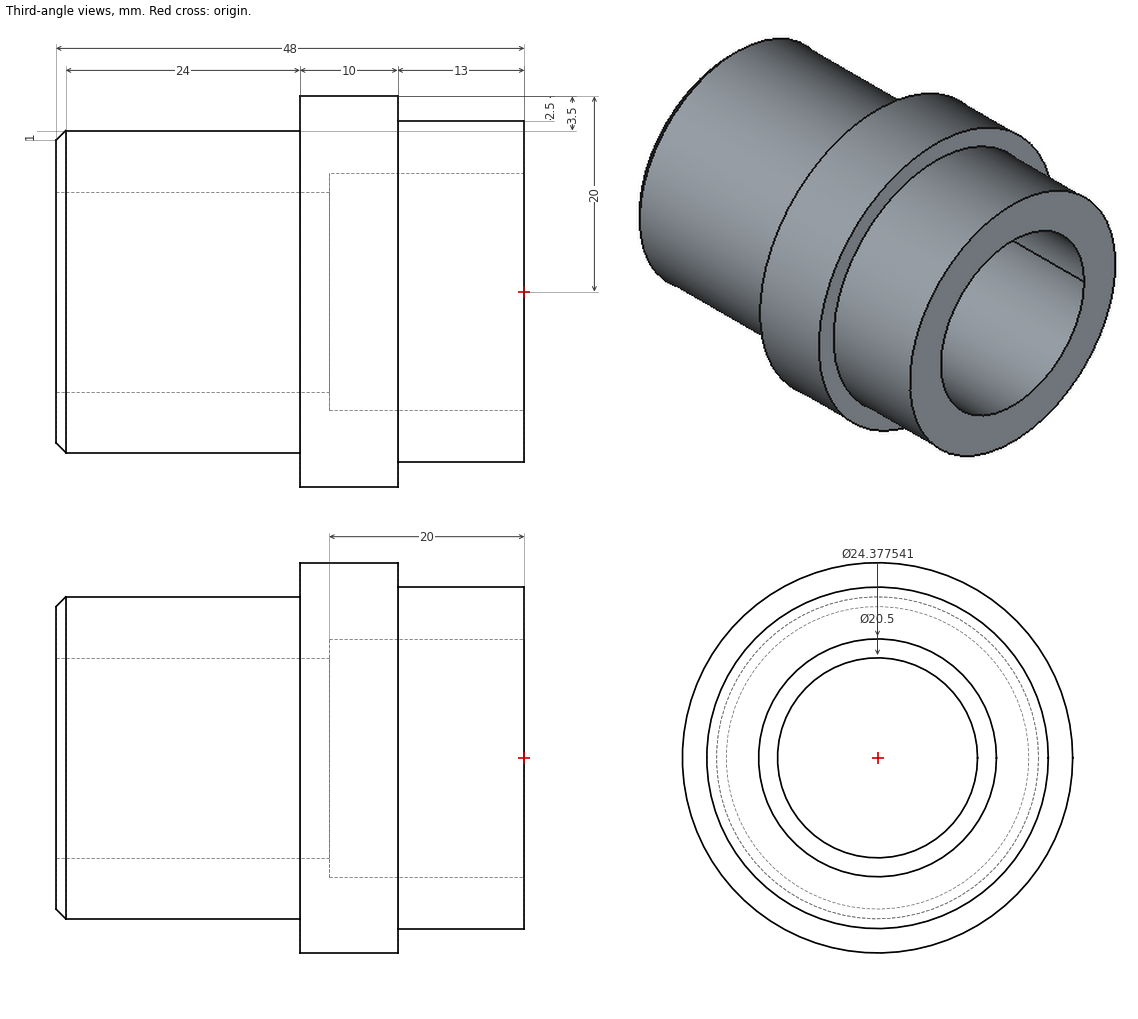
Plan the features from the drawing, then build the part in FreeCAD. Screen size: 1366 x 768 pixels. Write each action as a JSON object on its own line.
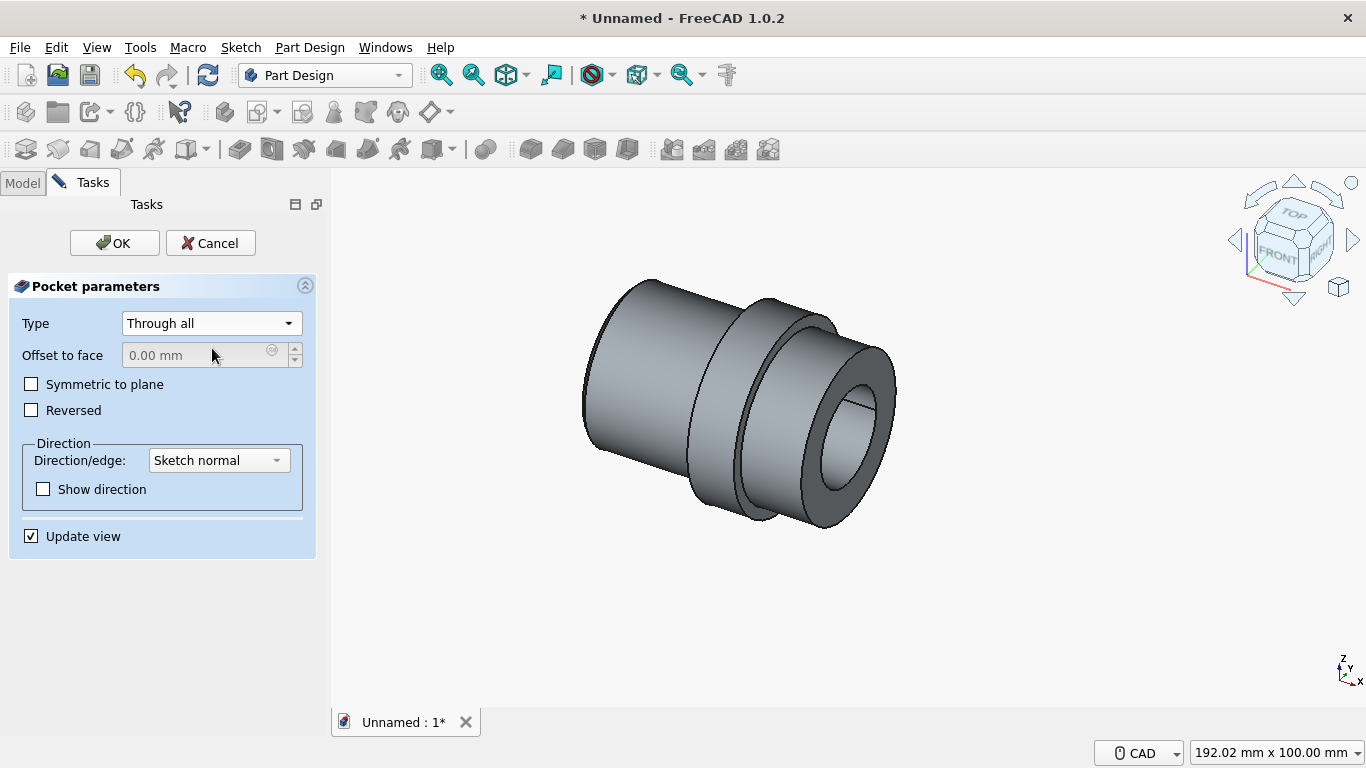
{"action": "left_click", "coordinate": [115, 243]}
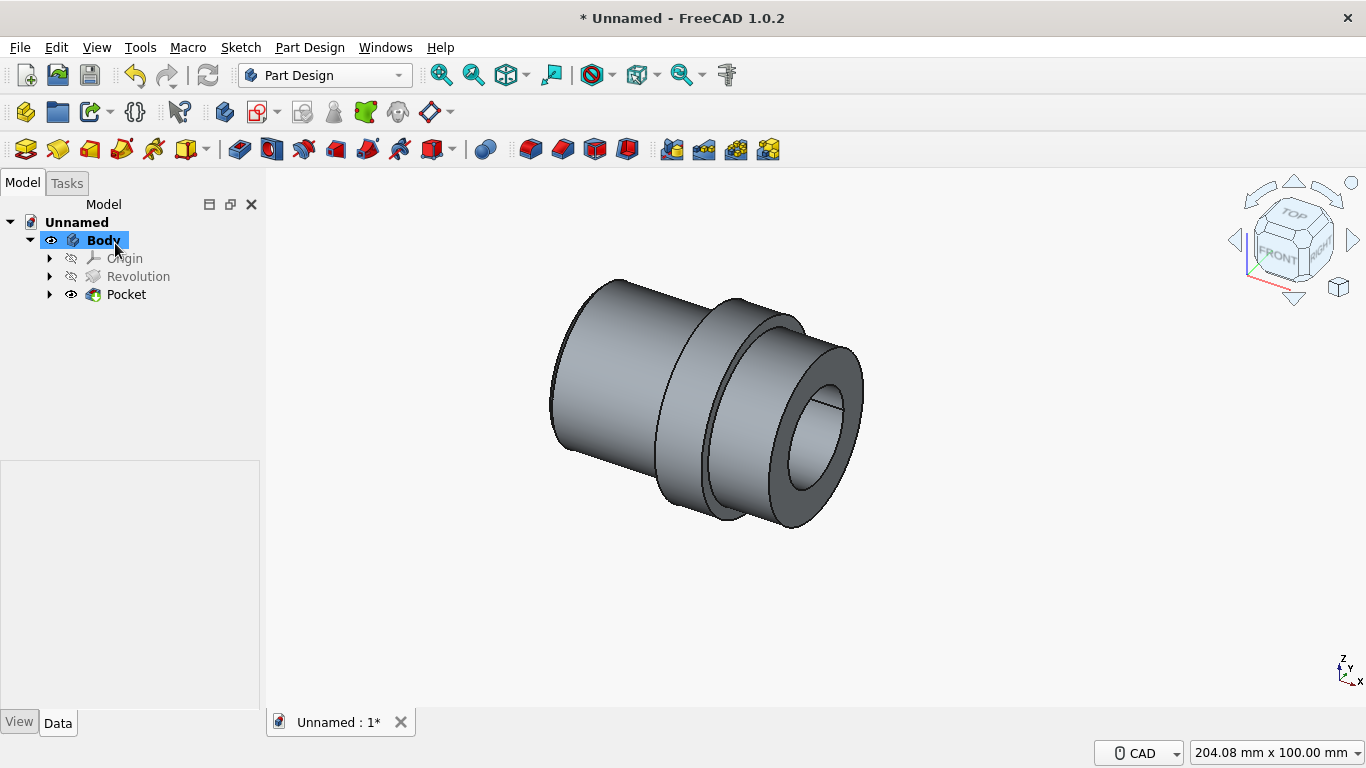
{"action": "left_click", "coordinate": [789, 507]}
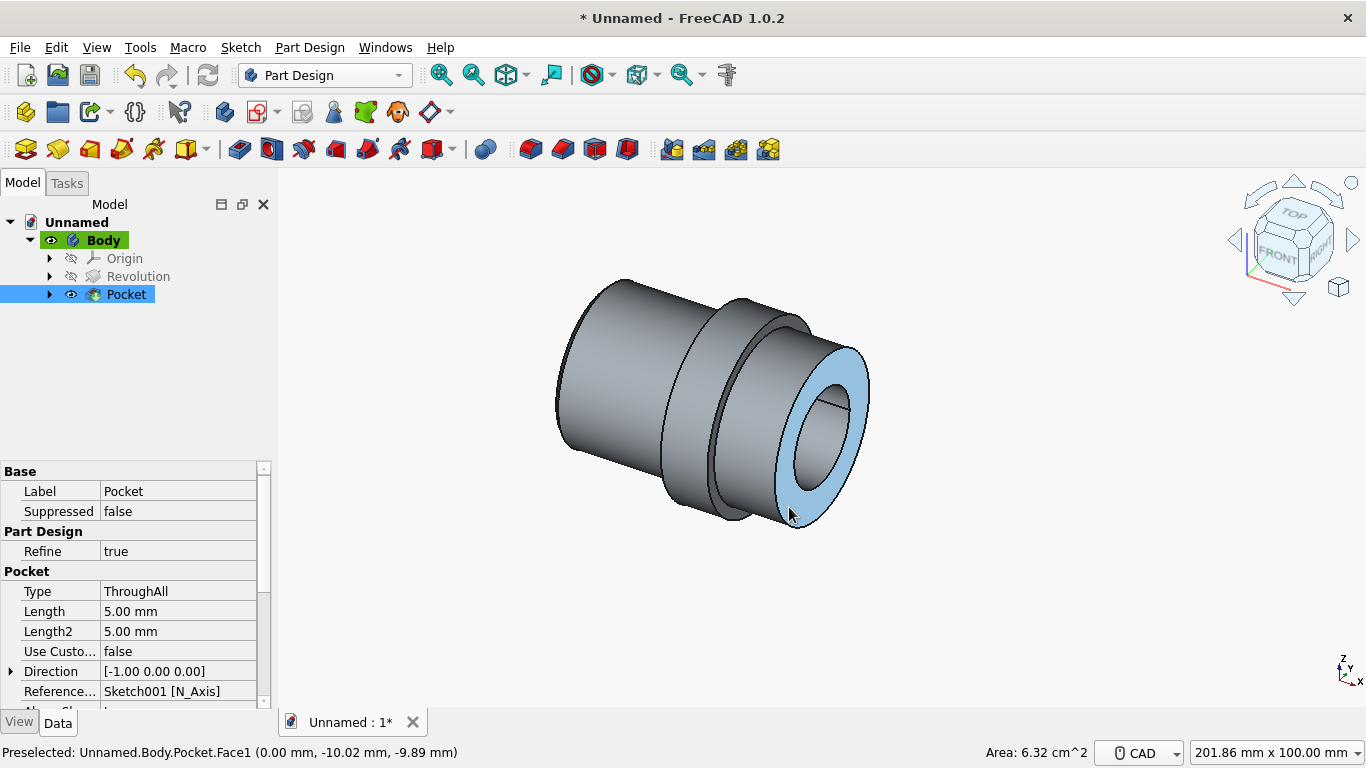
{"action": "left_click", "coordinate": [258, 112]}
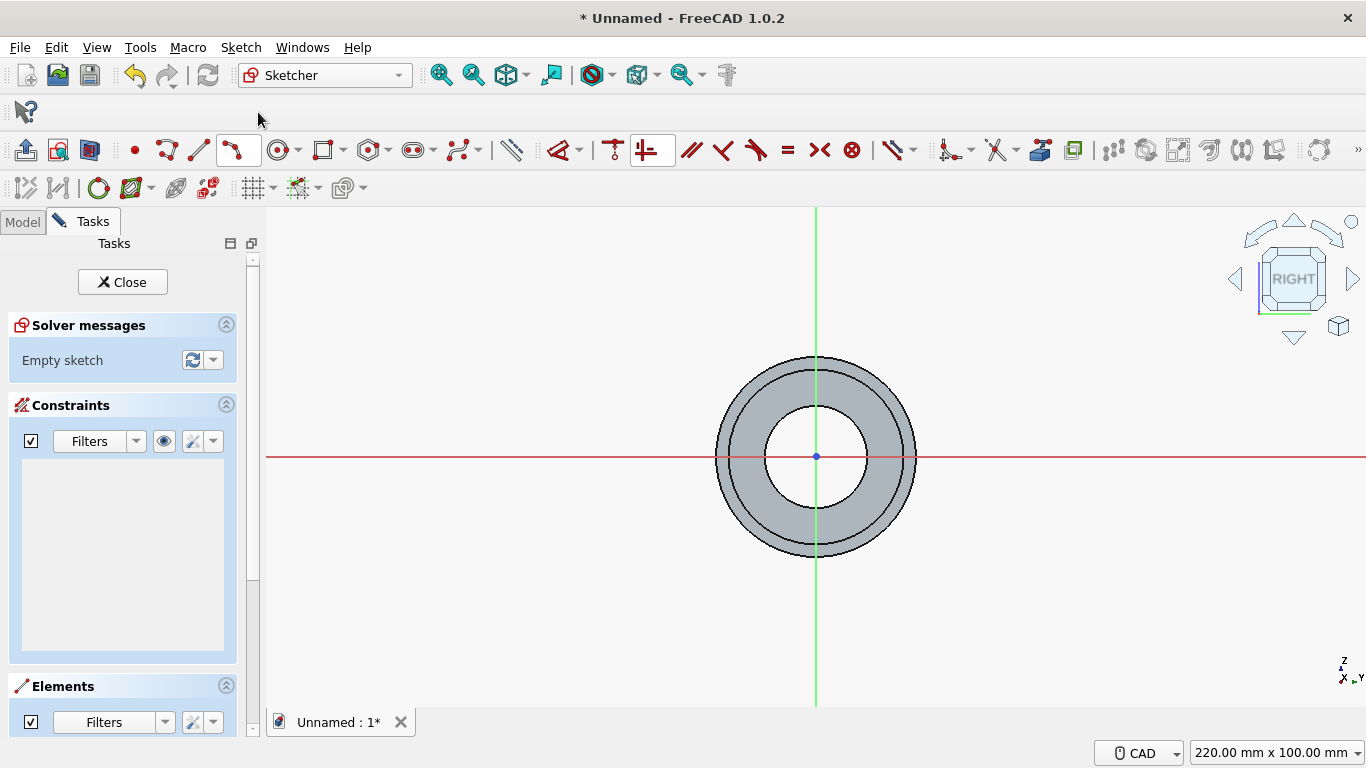
{"action": "scroll", "coordinate": [856, 457], "scroll_direction": "up", "scroll_amount": 5}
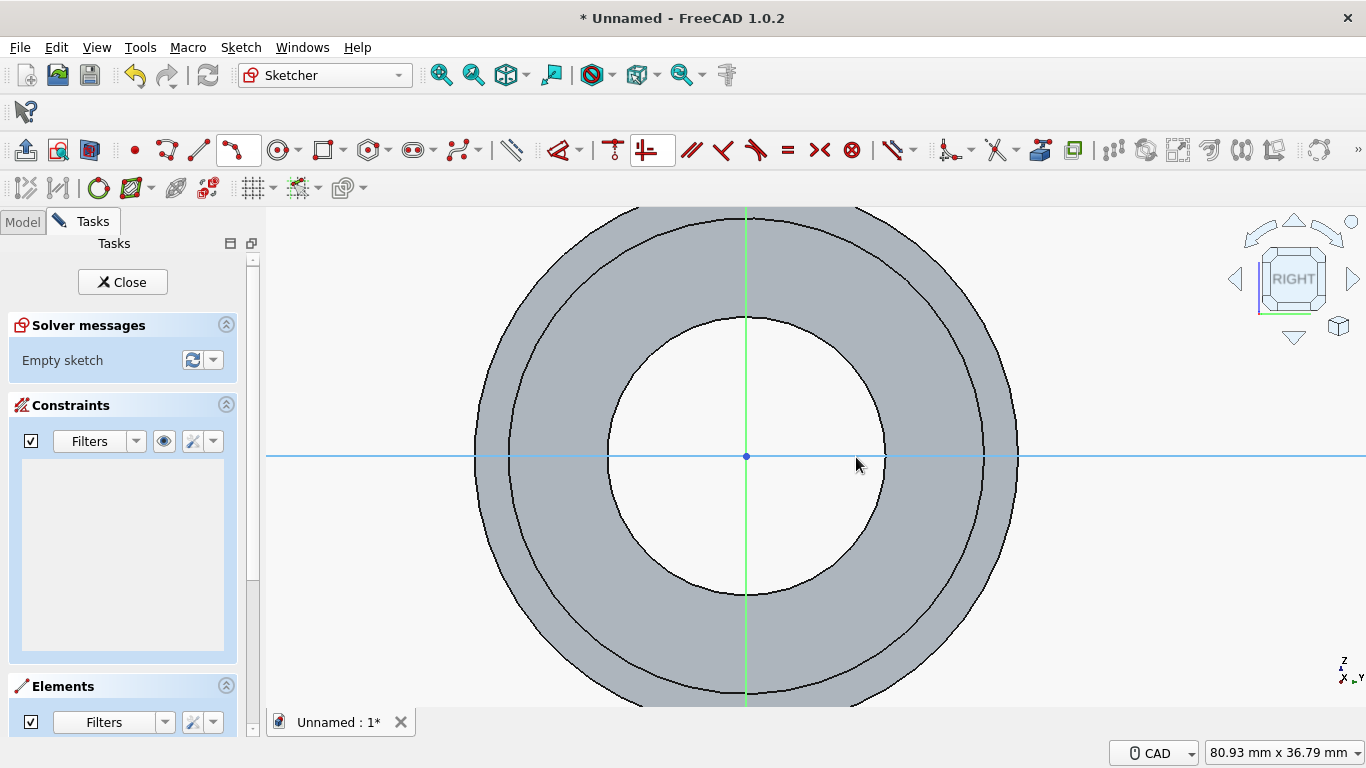
{"action": "left_click", "coordinate": [278, 150]}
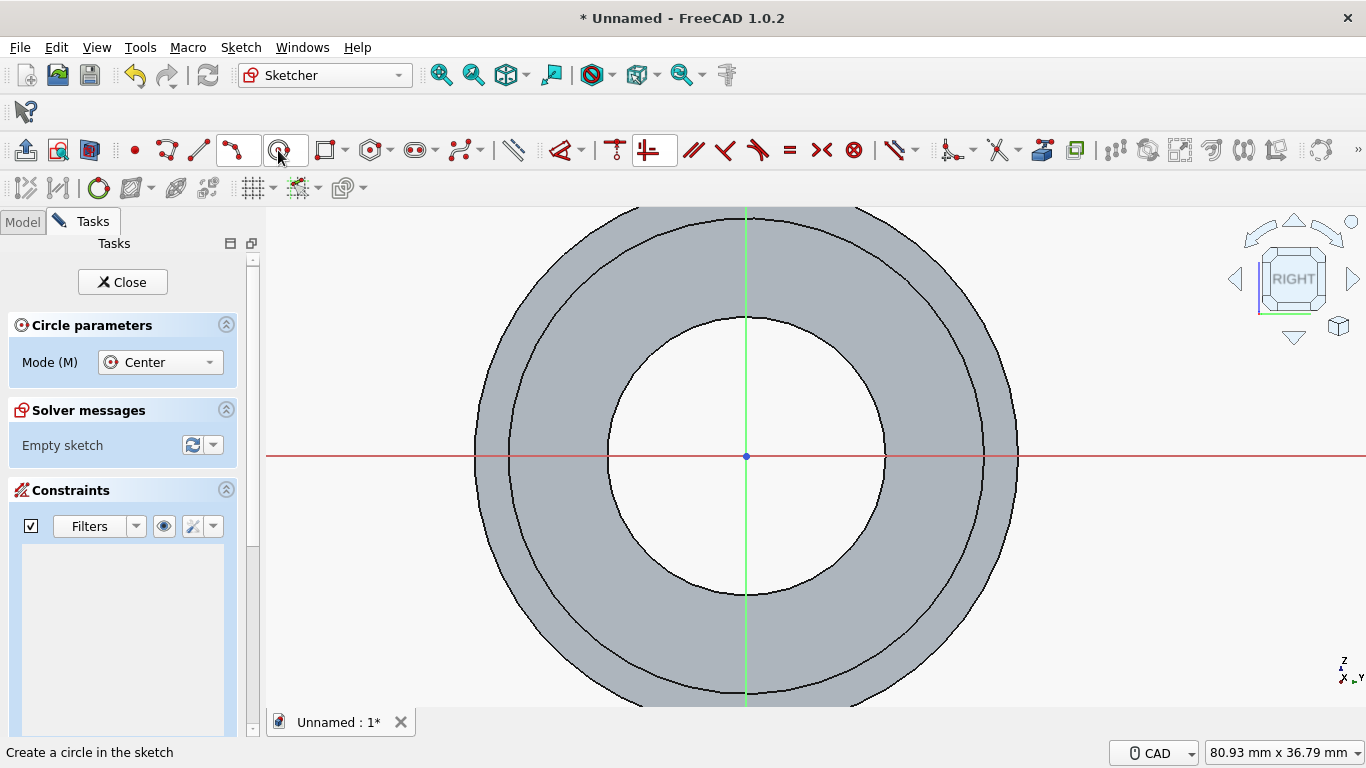
{"action": "left_click", "coordinate": [746, 456]}
{"action": "mouse_move", "coordinate": [863, 339]}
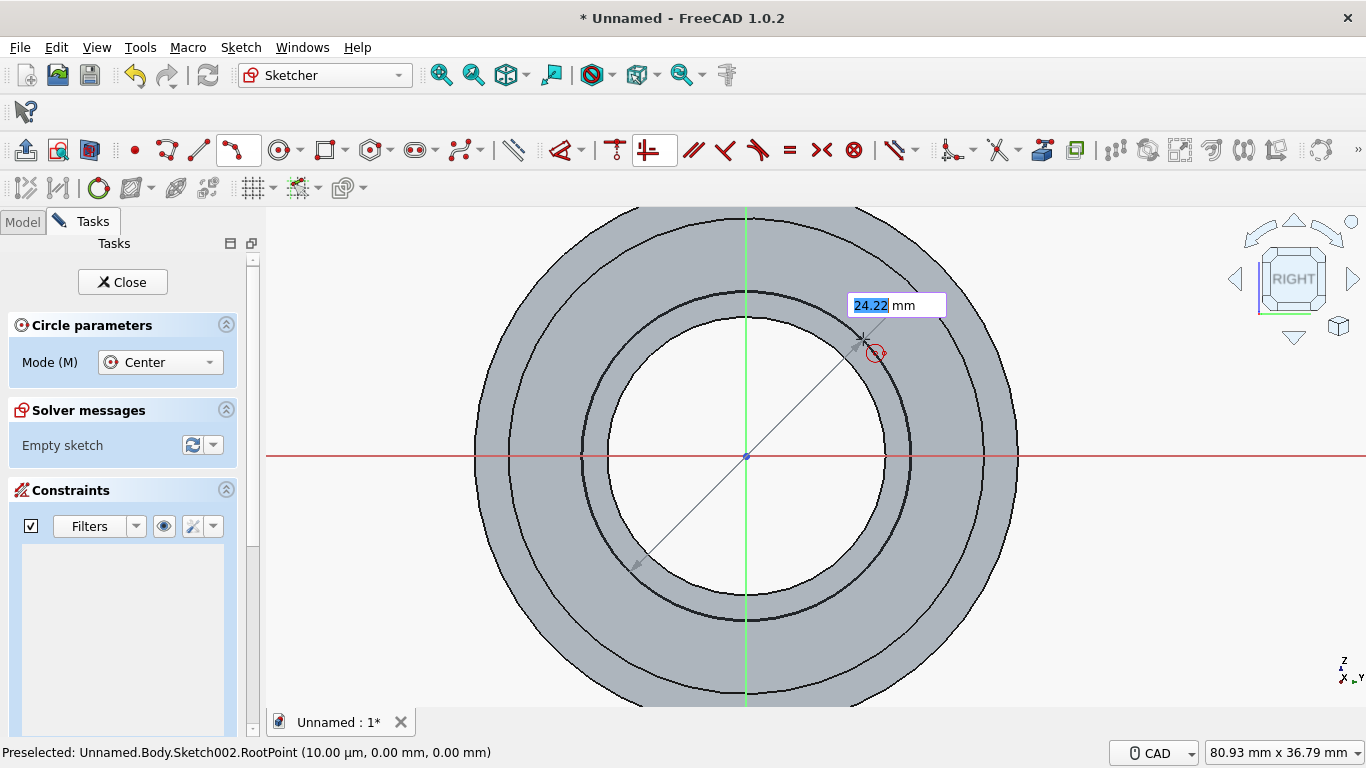
{"action": "type", "text": "24.377541"}
{"action": "key", "text": "Return"}
{"action": "key", "text": "Escape"}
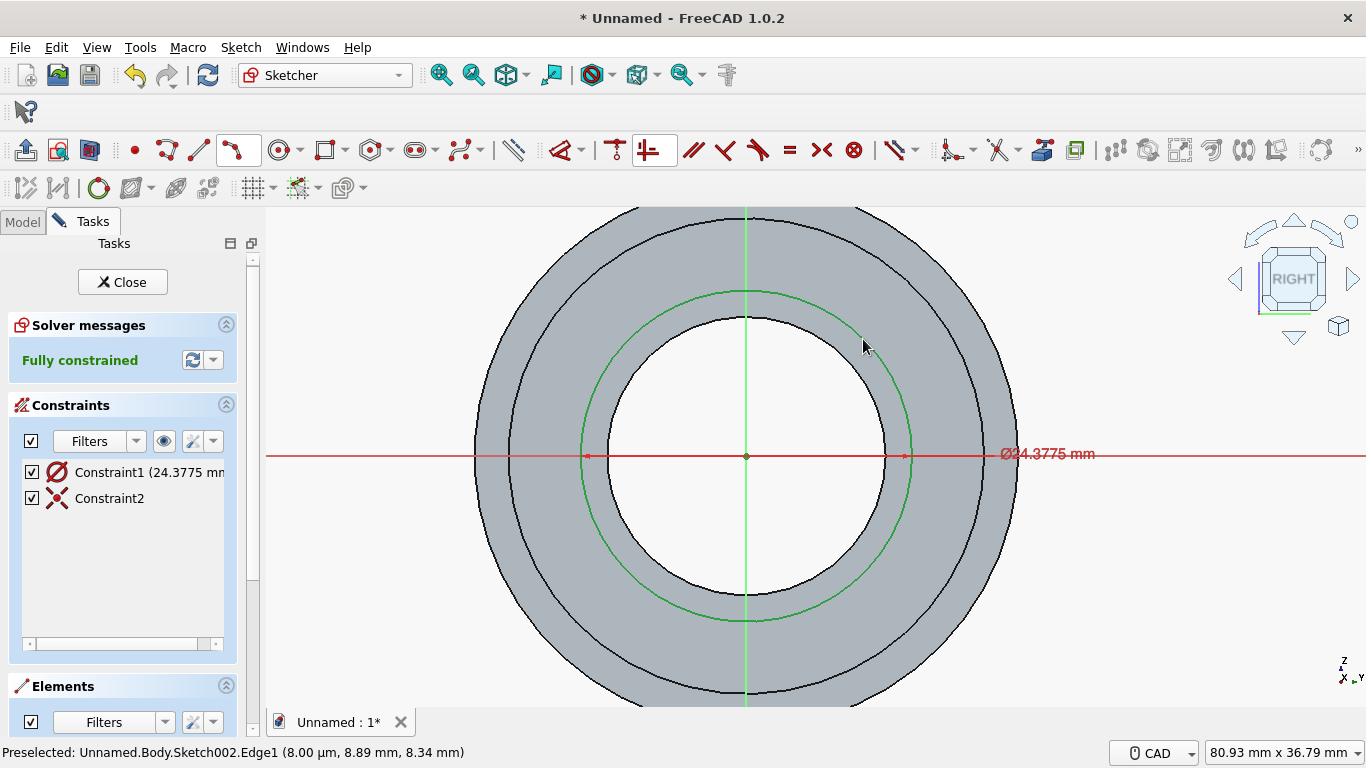
{"action": "left_click", "coordinate": [123, 282]}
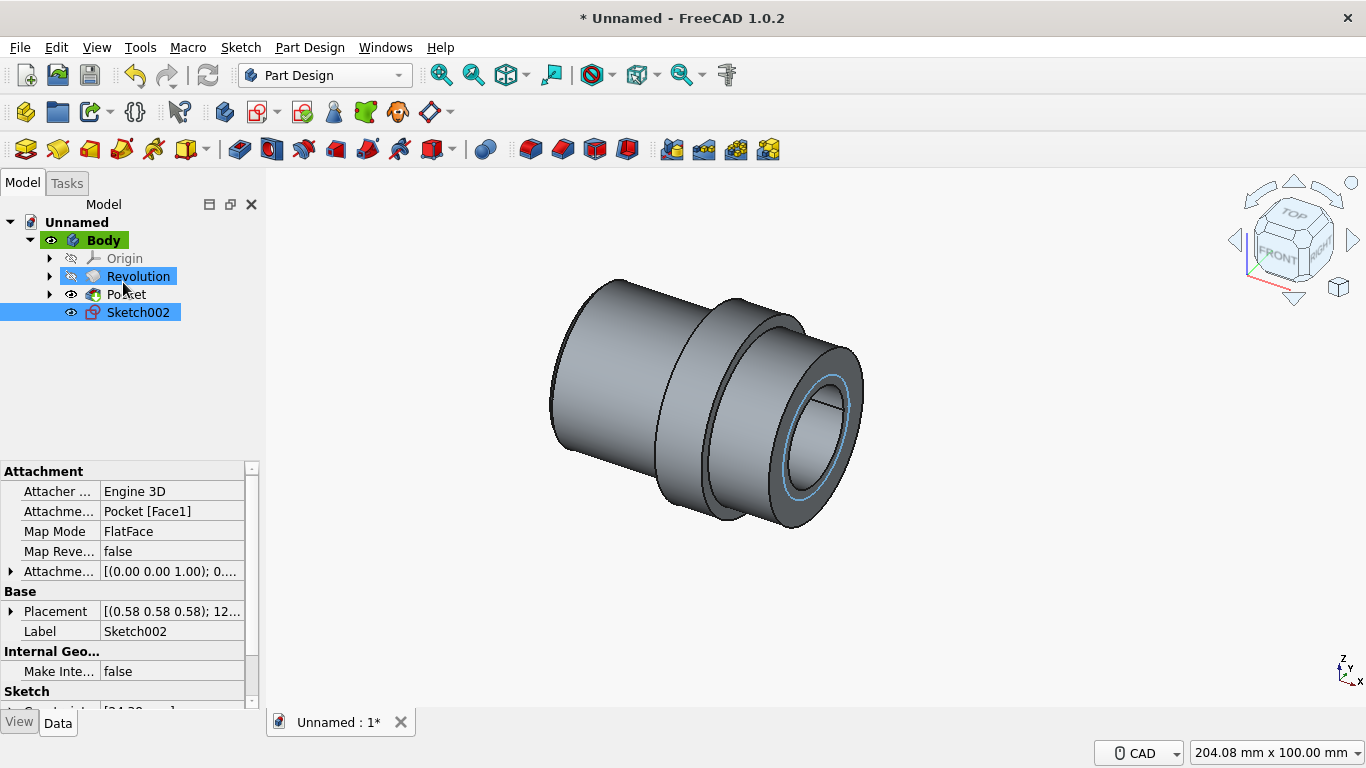
{"action": "left_click", "coordinate": [240, 150]}